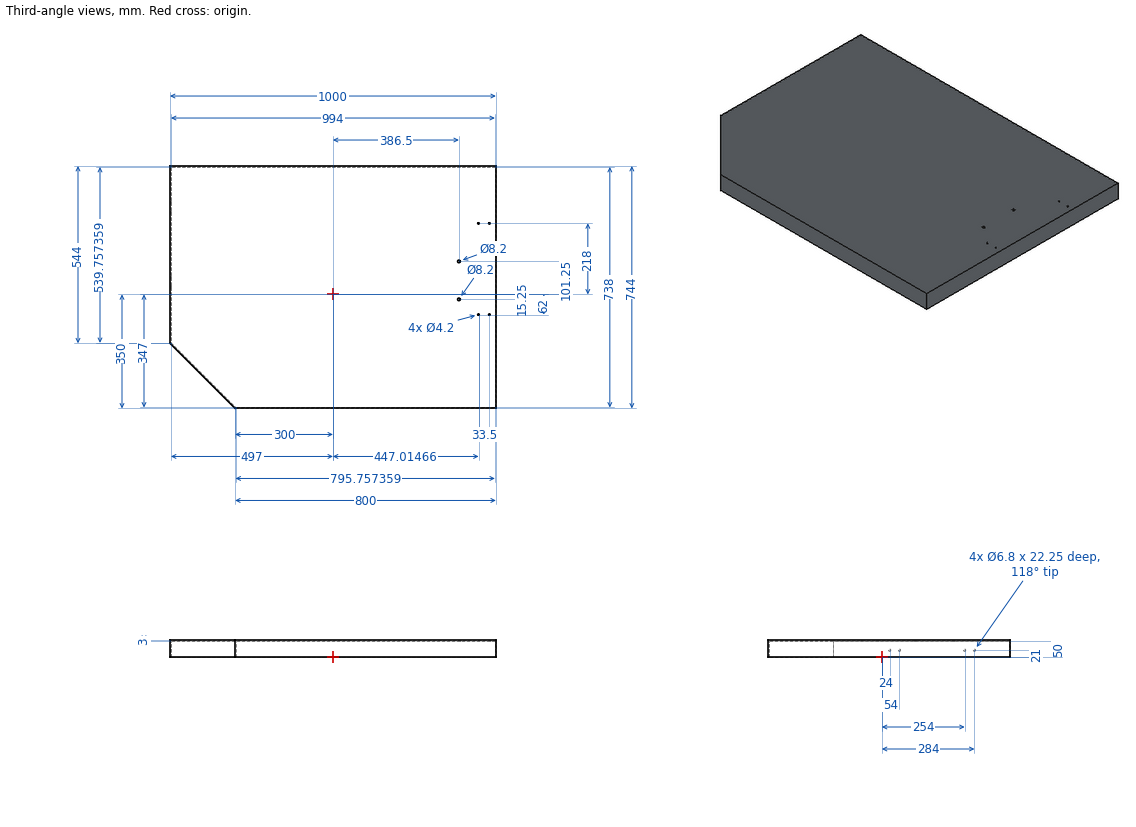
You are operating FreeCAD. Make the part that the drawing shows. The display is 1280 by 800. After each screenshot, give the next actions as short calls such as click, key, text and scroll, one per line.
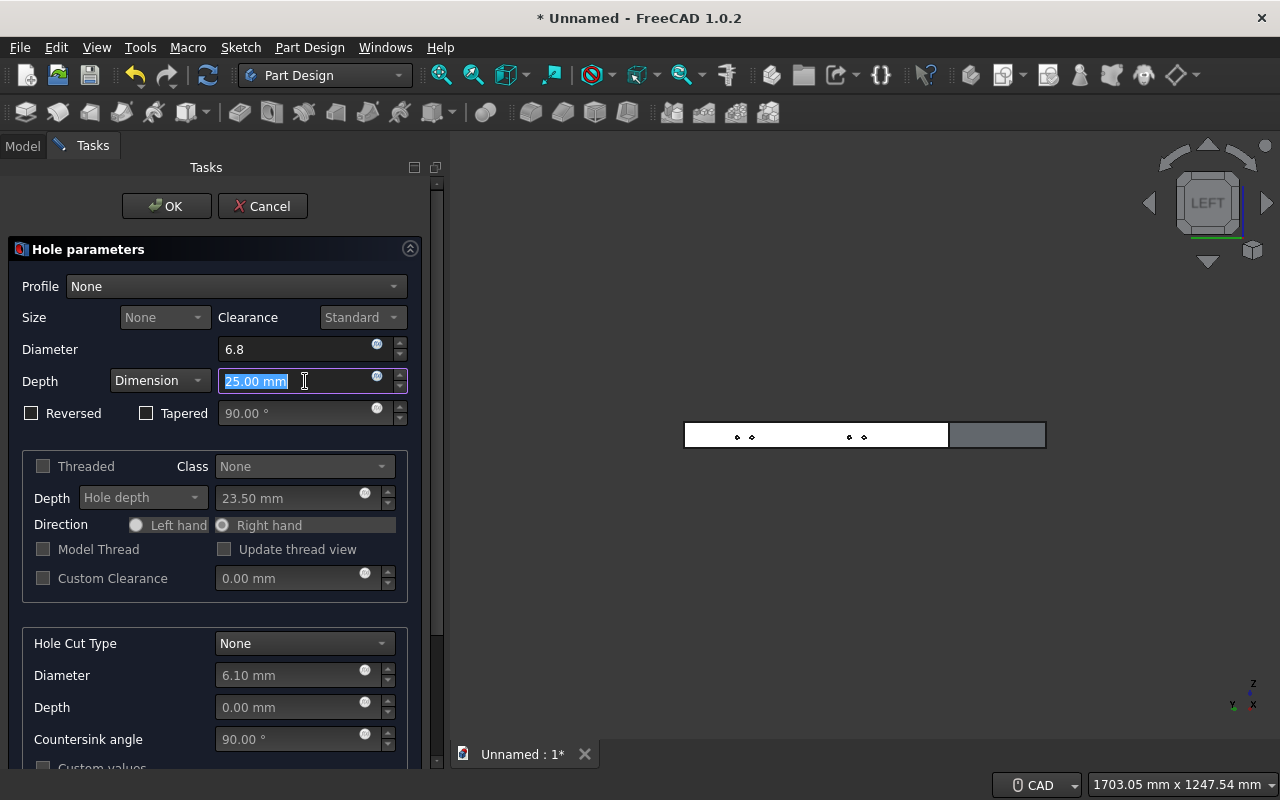
text(22.25)
key(Tab)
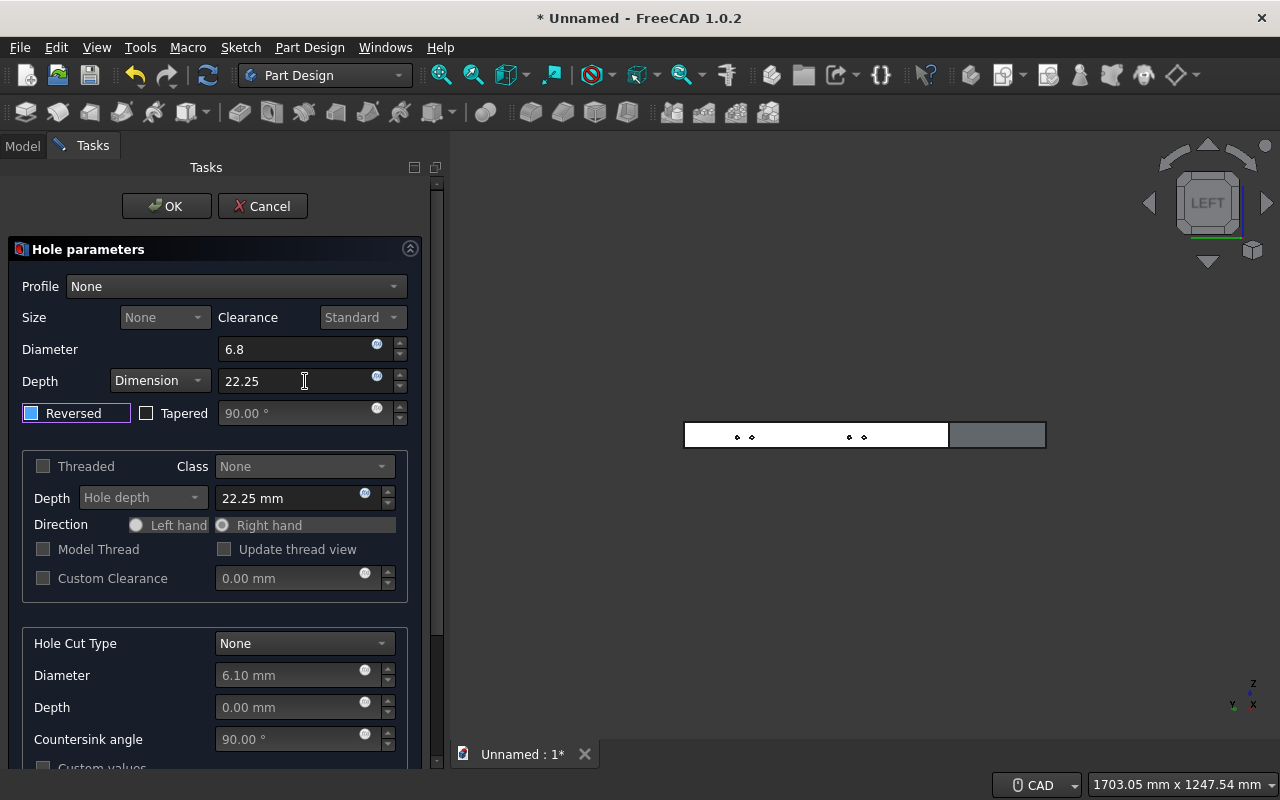
click(167, 206)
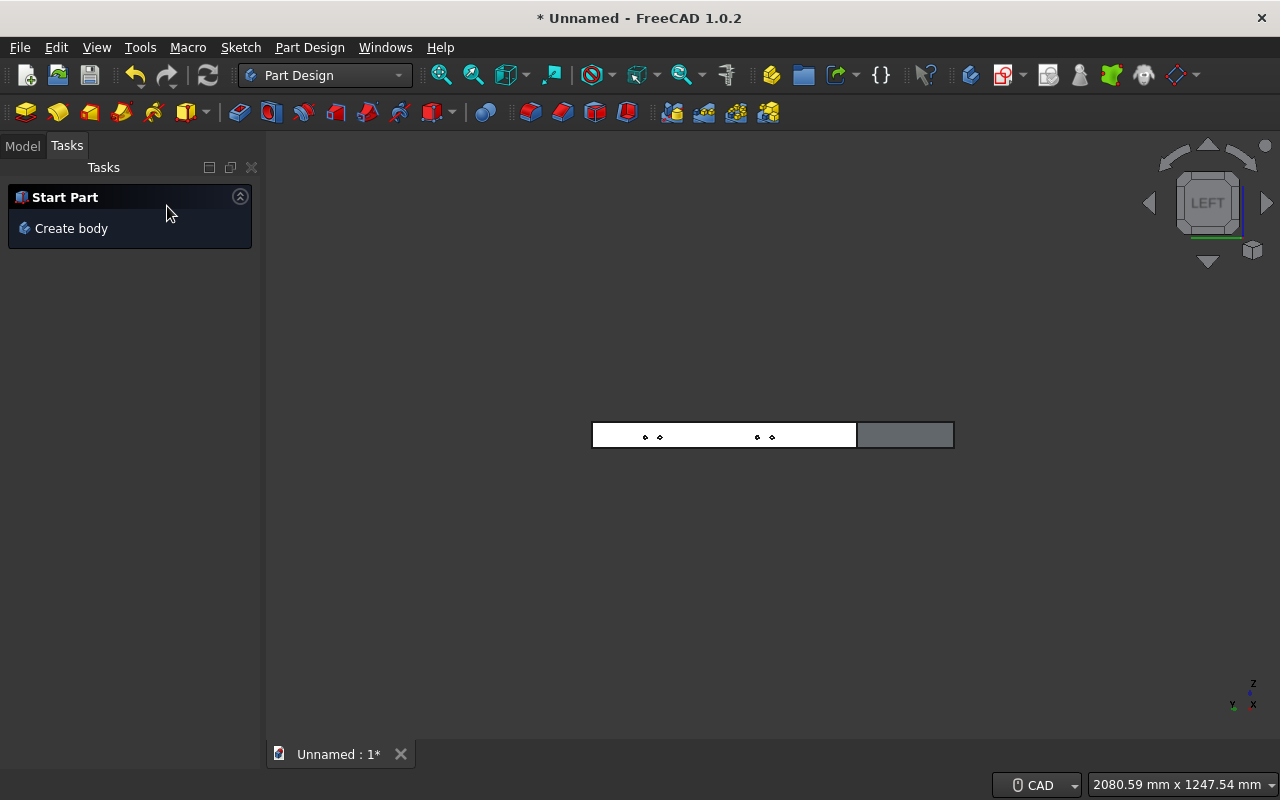
click(442, 76)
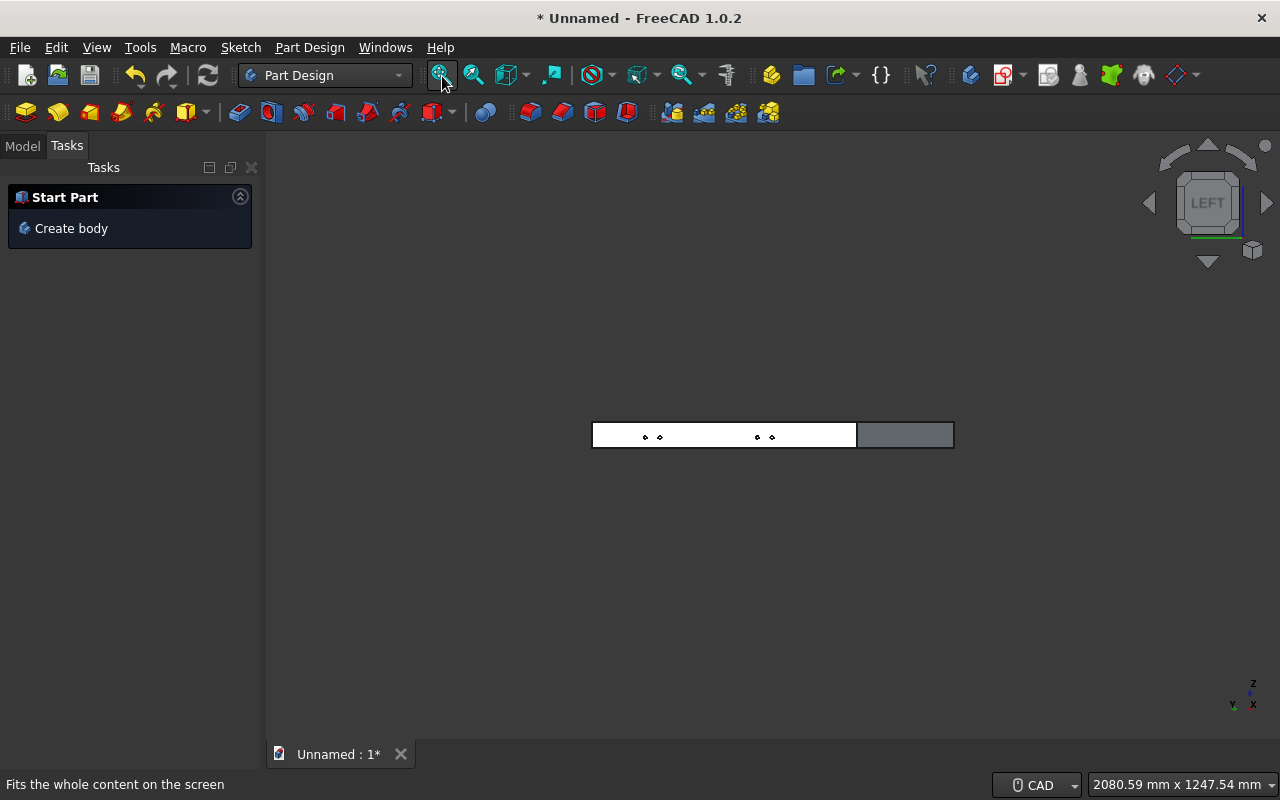
key(0)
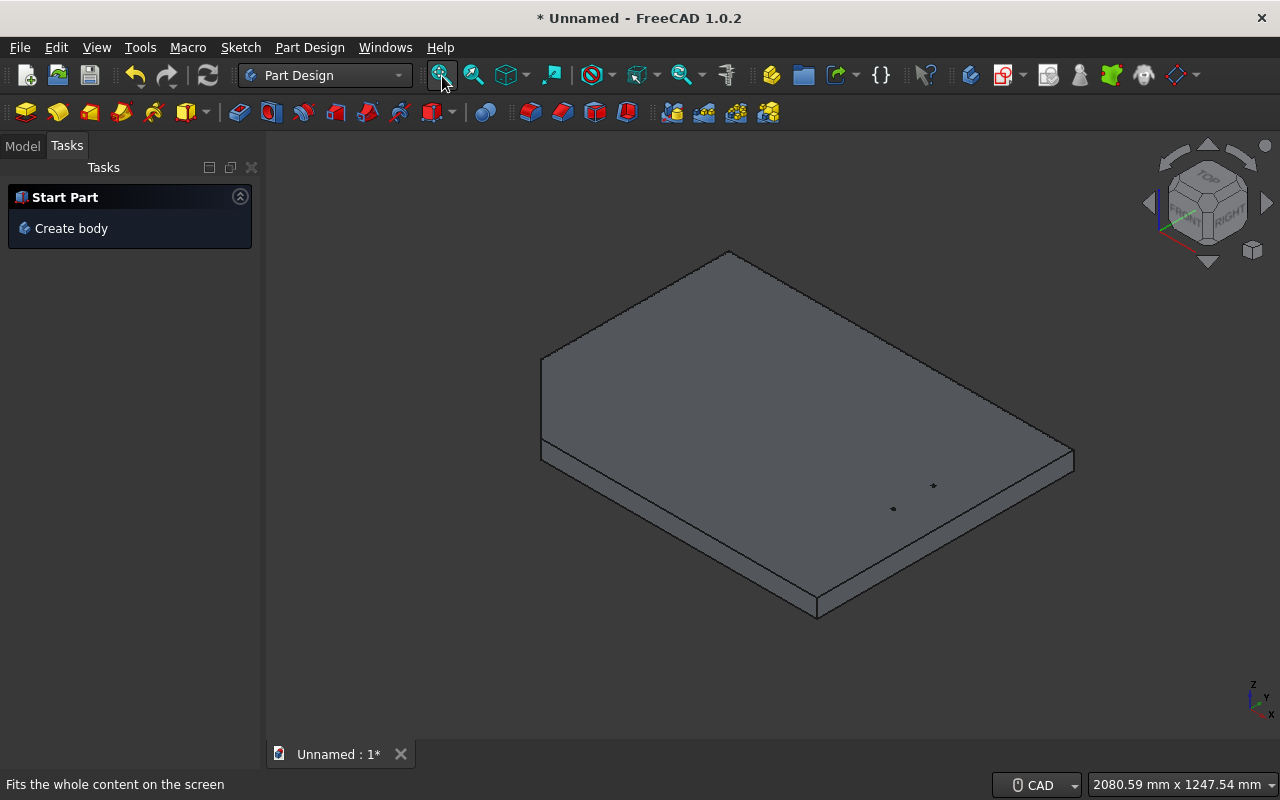
click(773, 423)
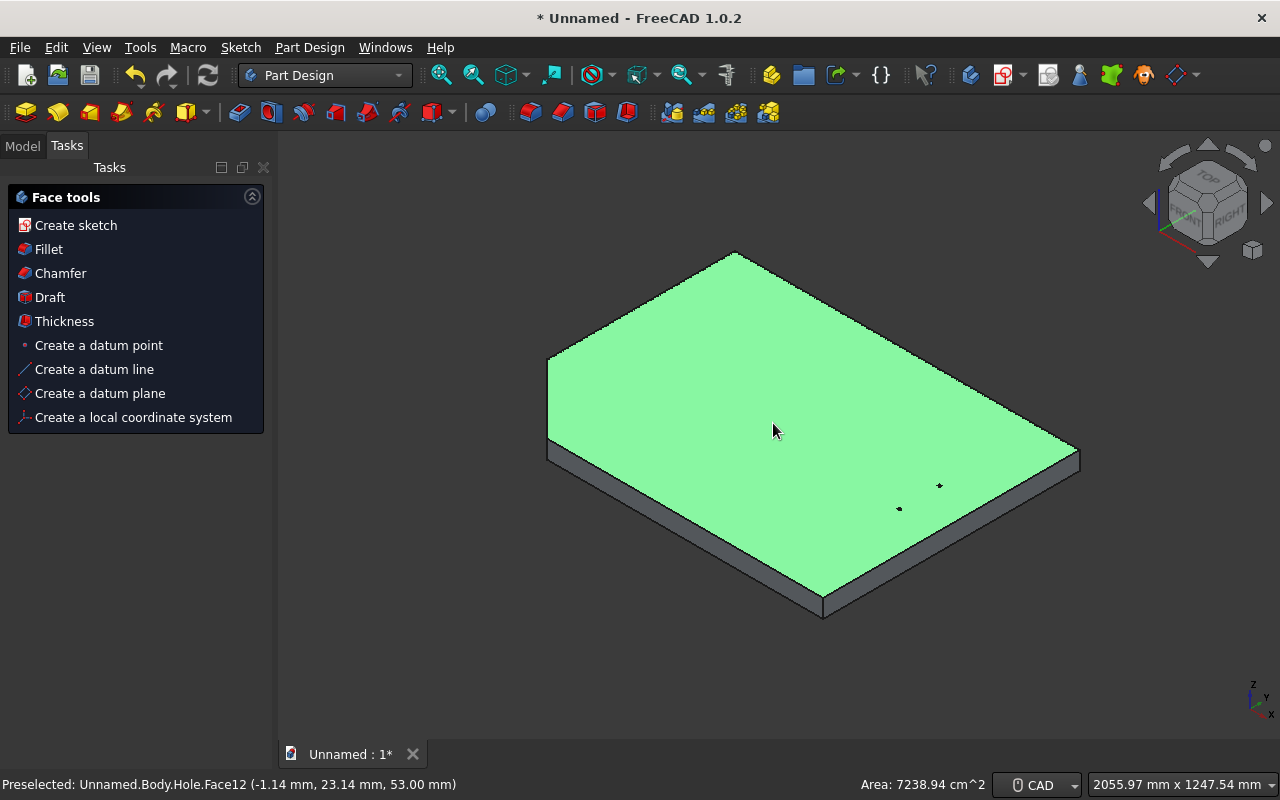
click(1004, 76)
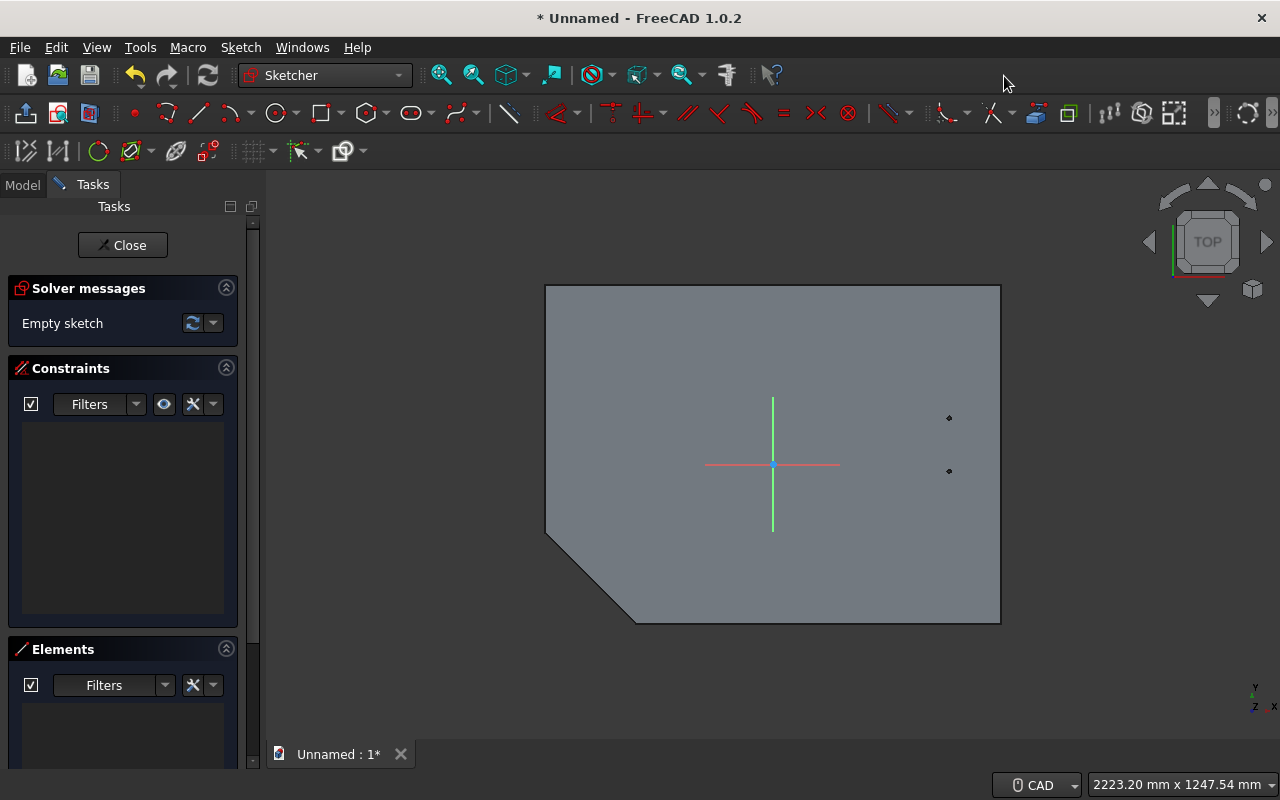
scroll(987, 414, up, 5)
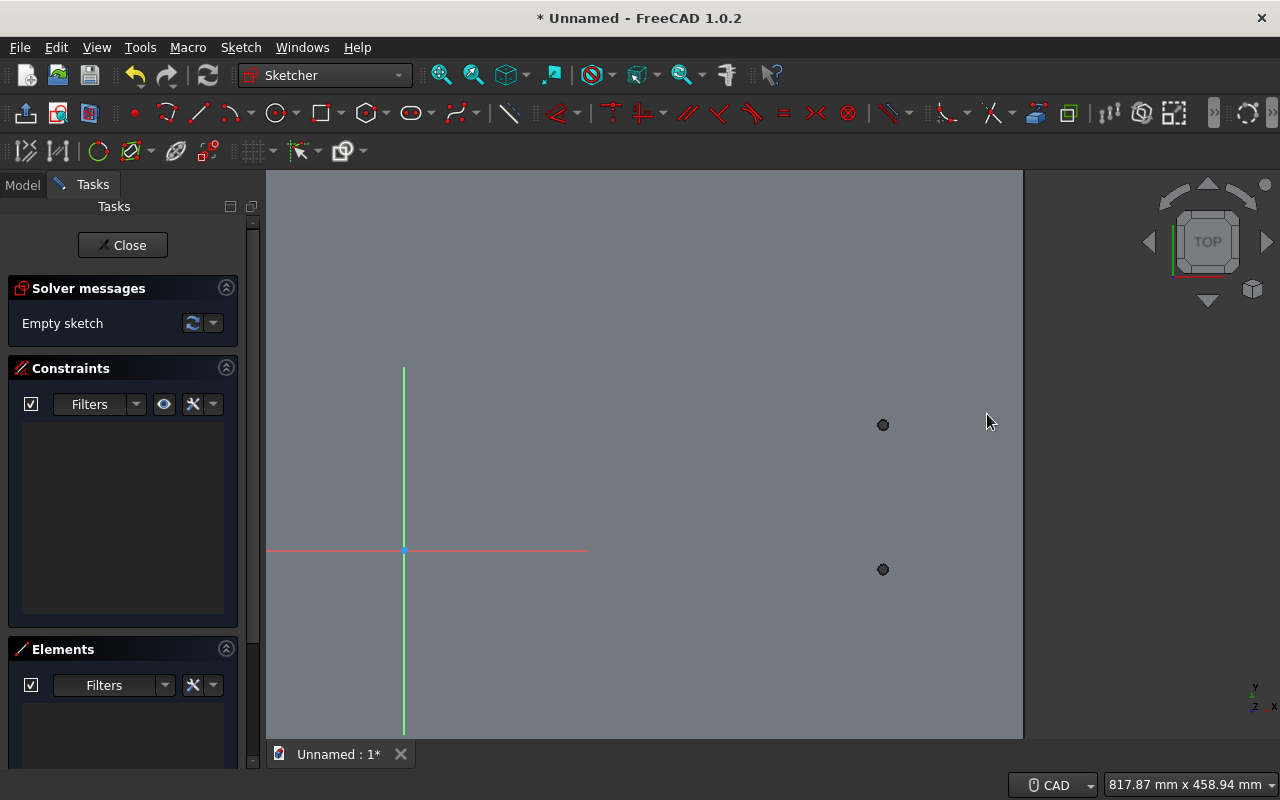
click(276, 114)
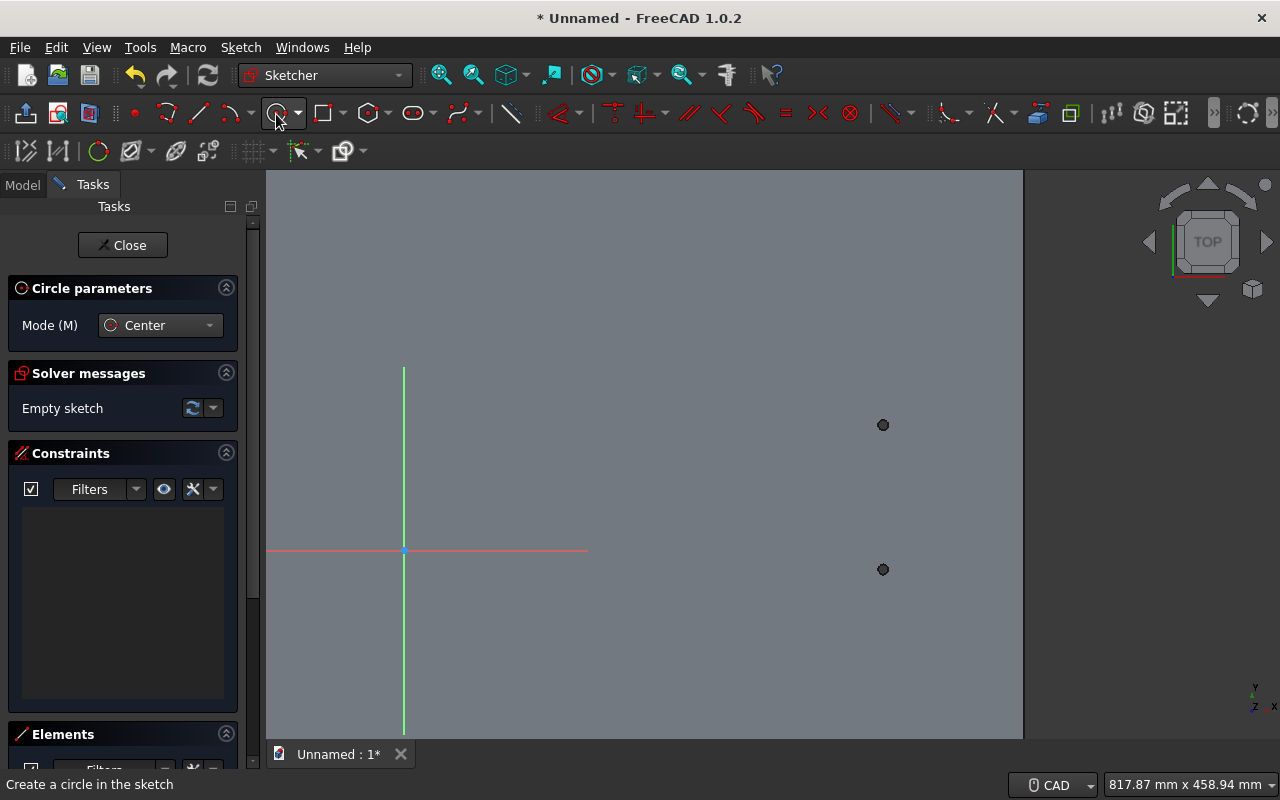
scroll(958, 627, up, 11)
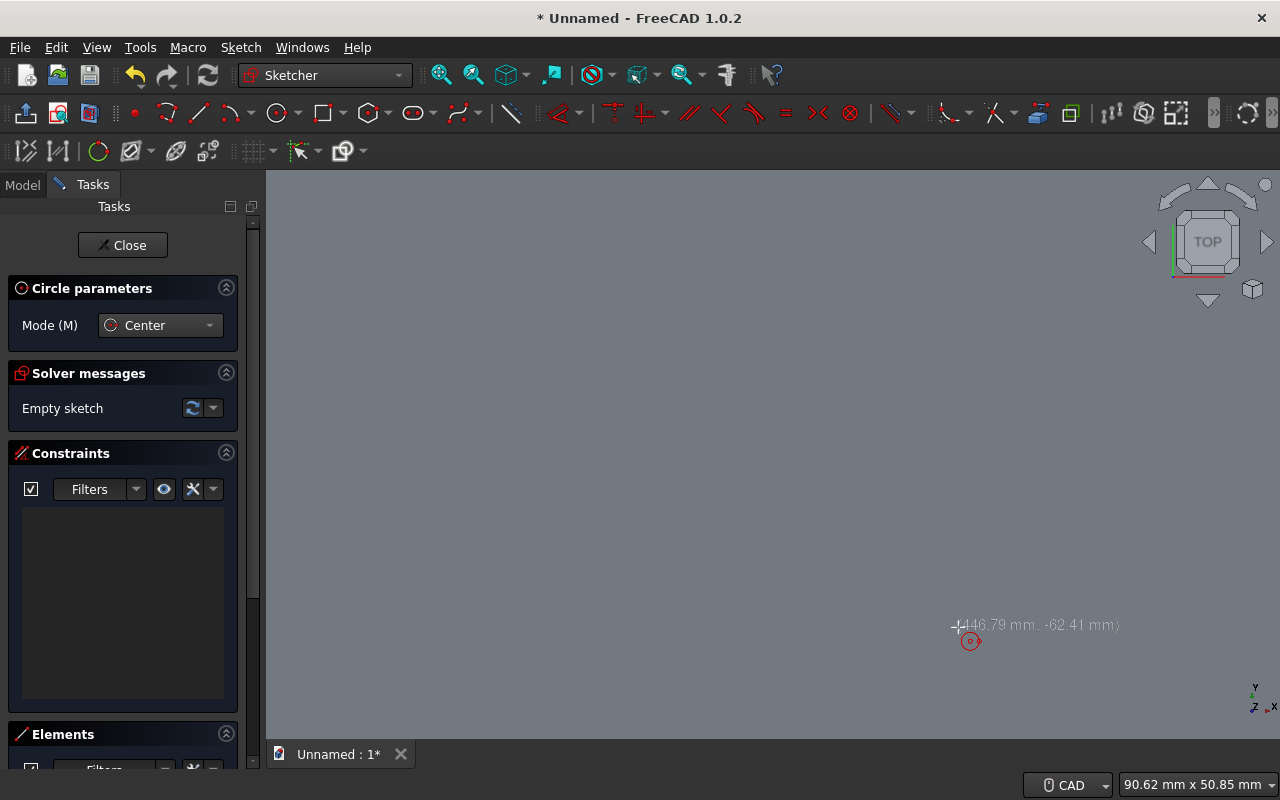
scroll(960, 628, down, 11)